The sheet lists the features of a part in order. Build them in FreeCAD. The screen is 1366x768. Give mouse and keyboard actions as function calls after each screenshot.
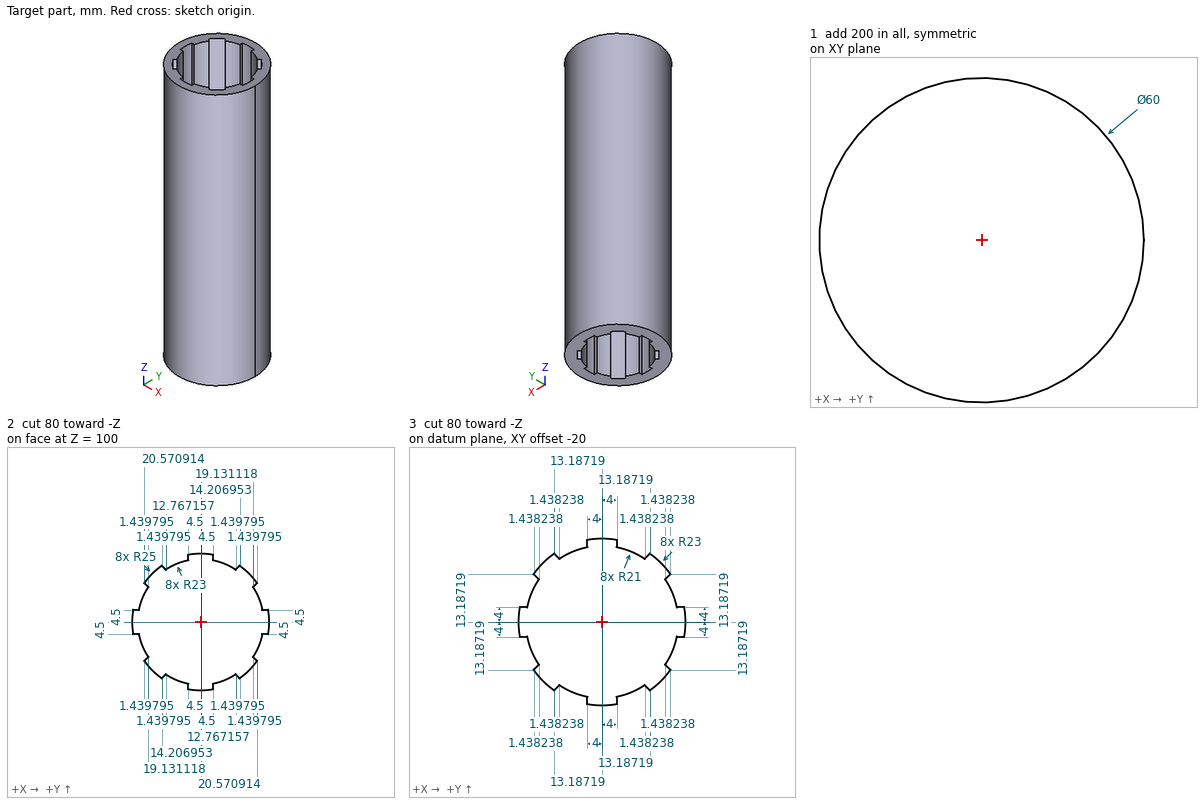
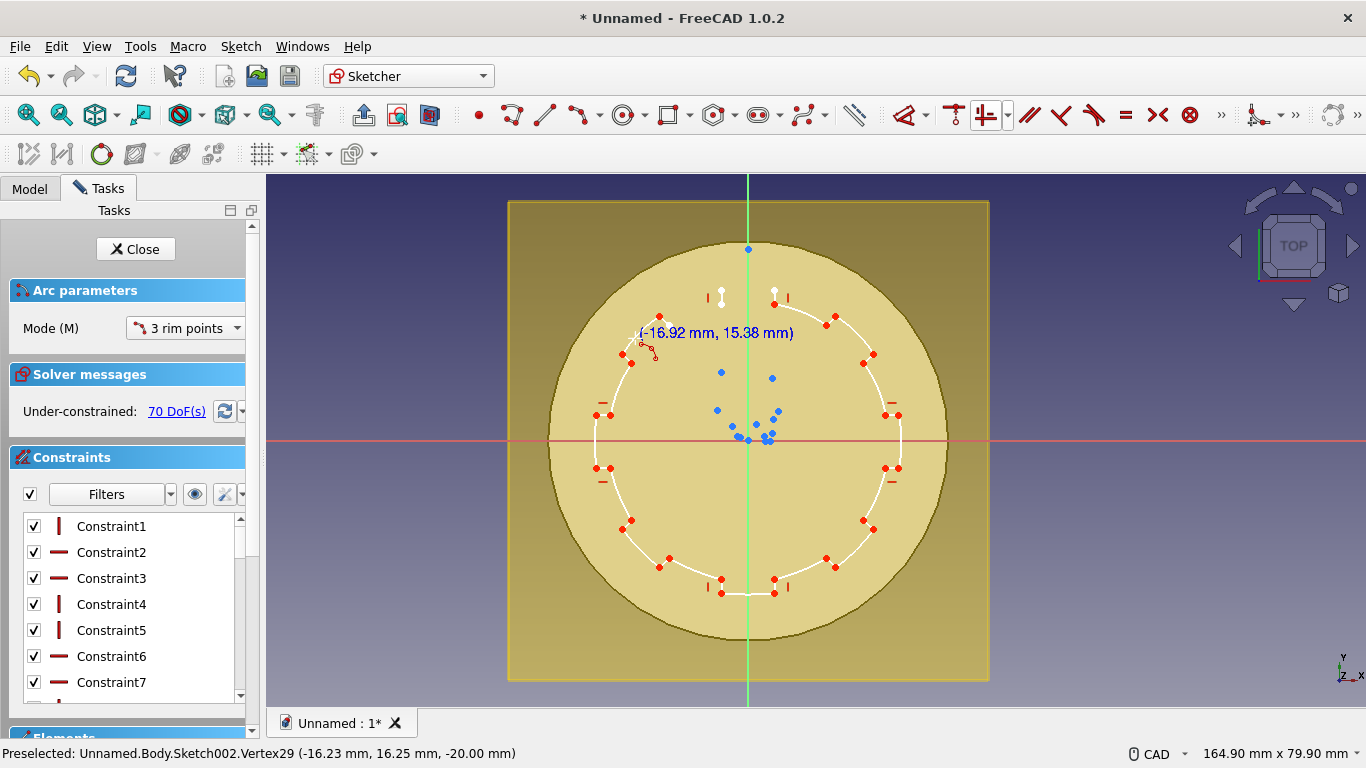
scroll(670, 325, up, 5)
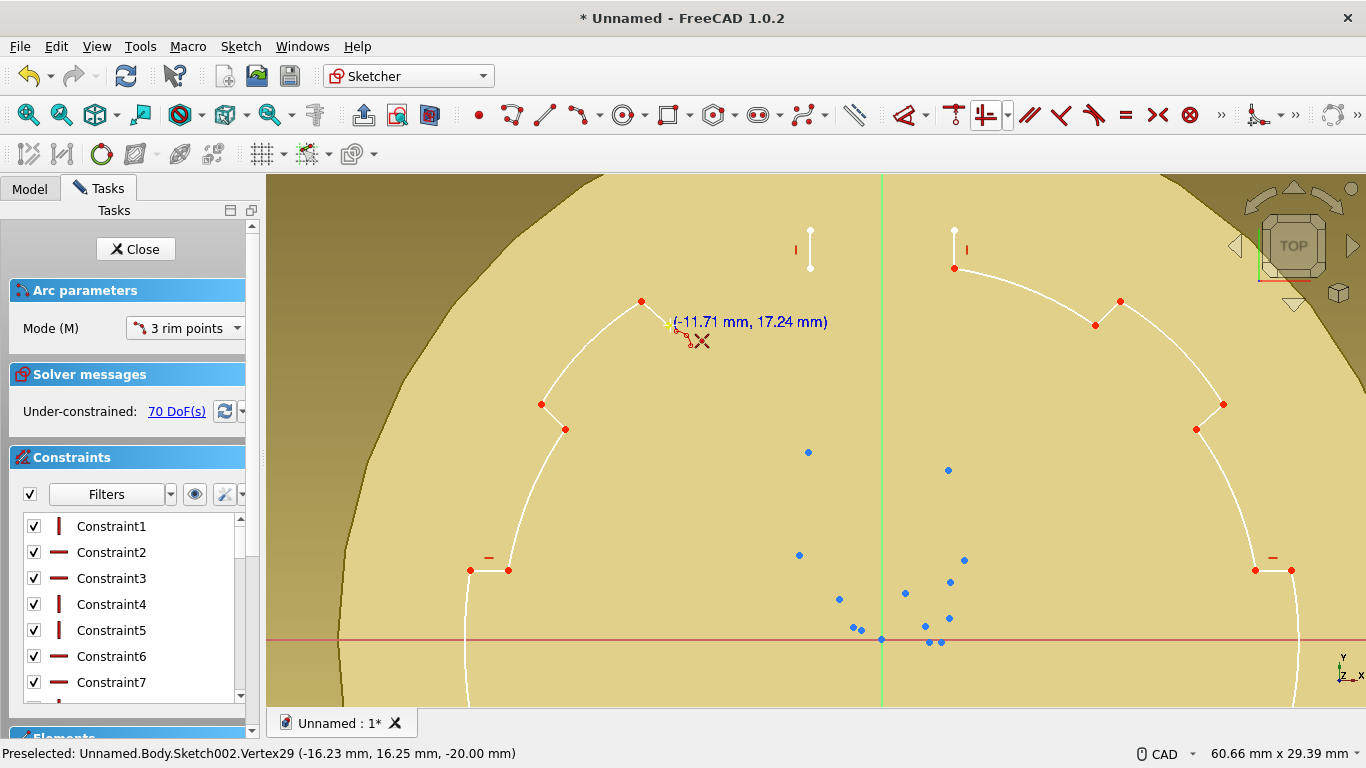
click(669, 326)
click(810, 269)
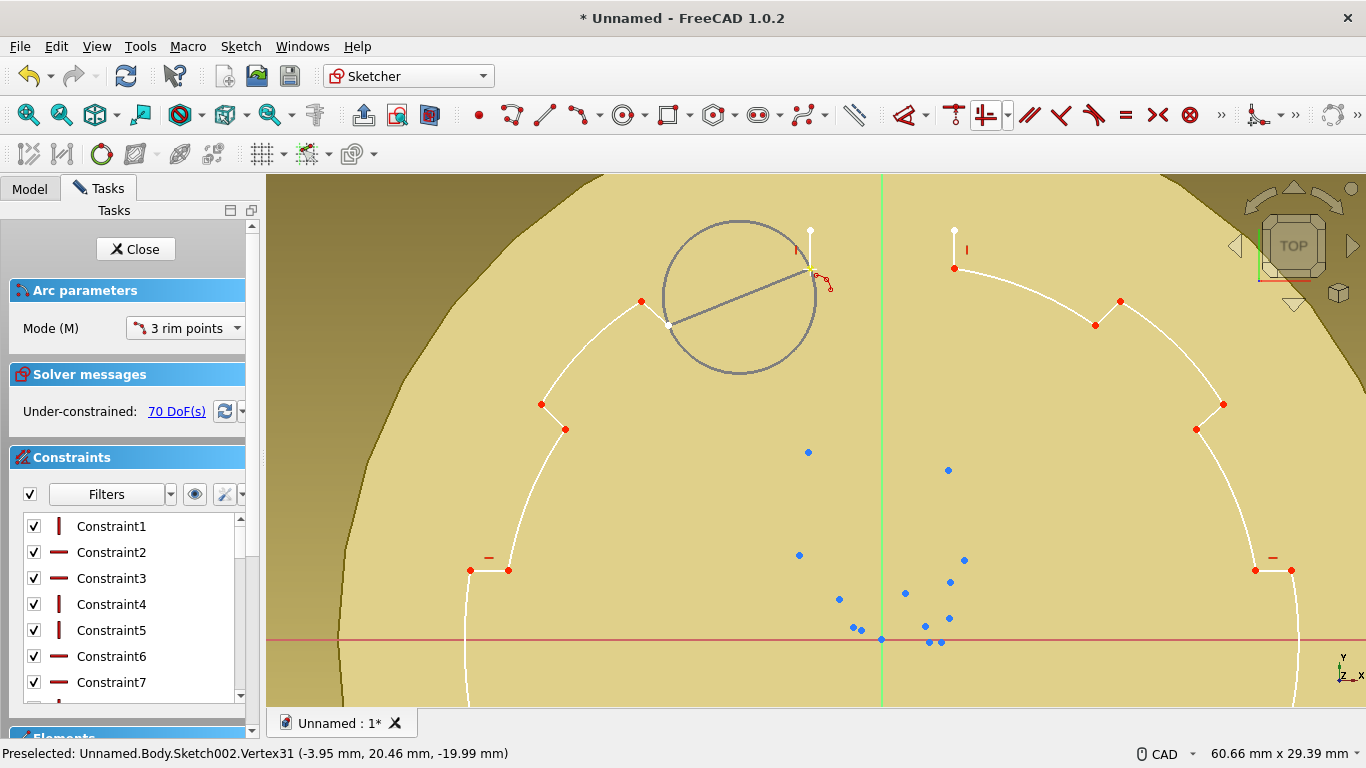
scroll(736, 288, up, 4)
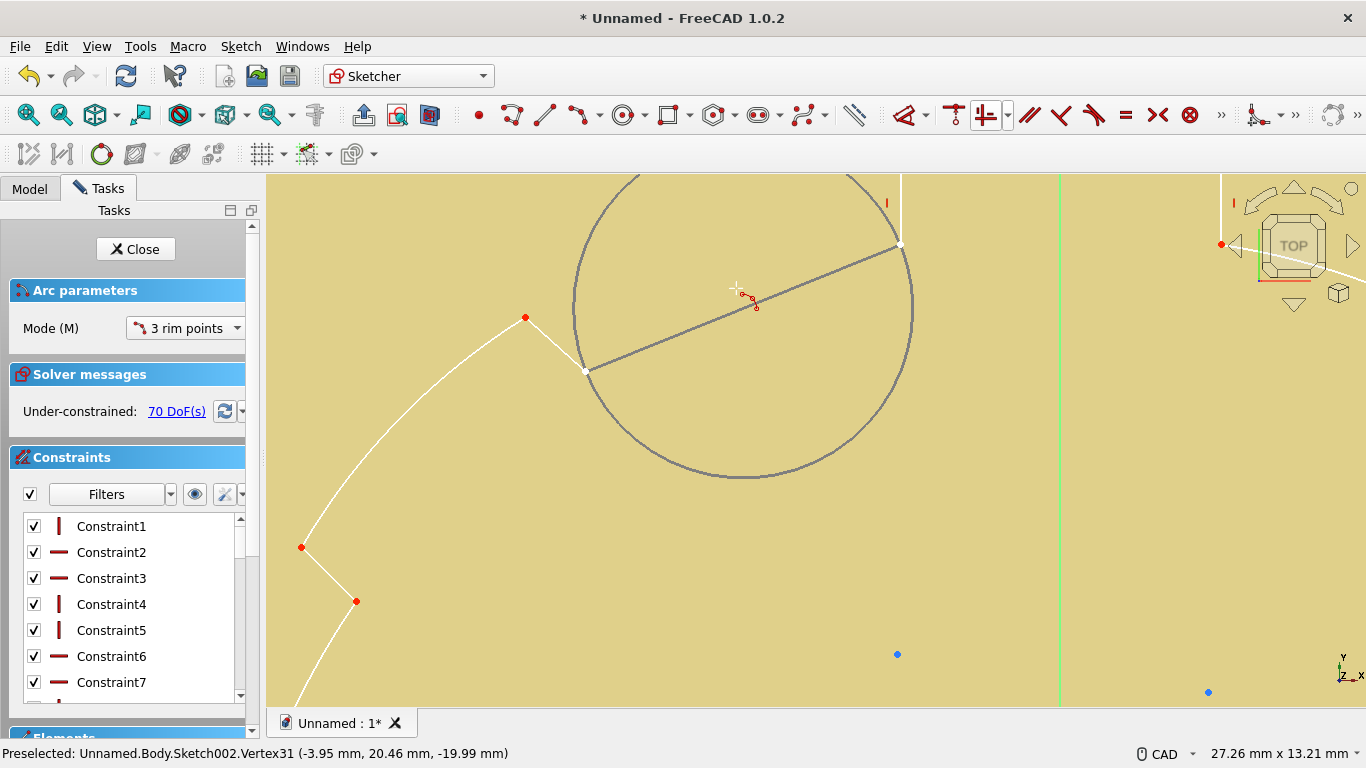
click(736, 288)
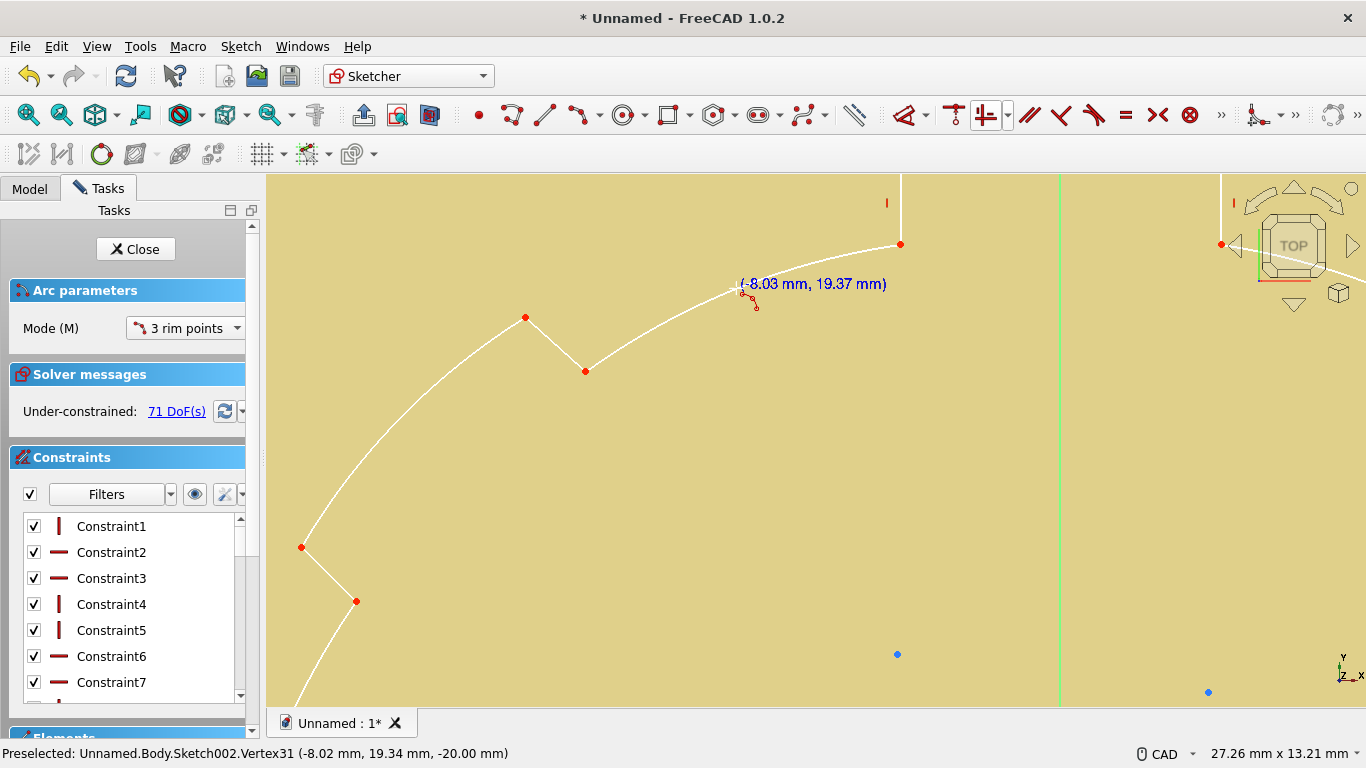
scroll(686, 316, down, 9)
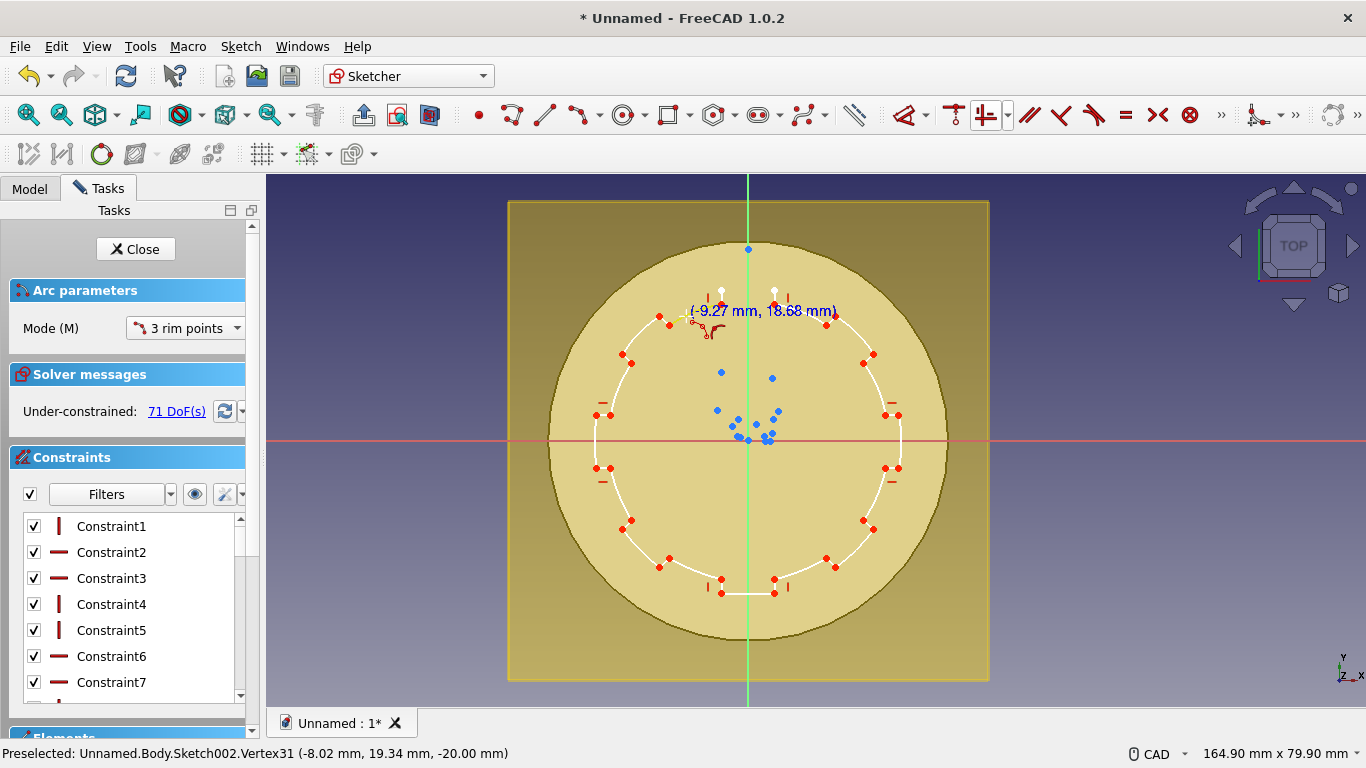
scroll(721, 290, up, 5)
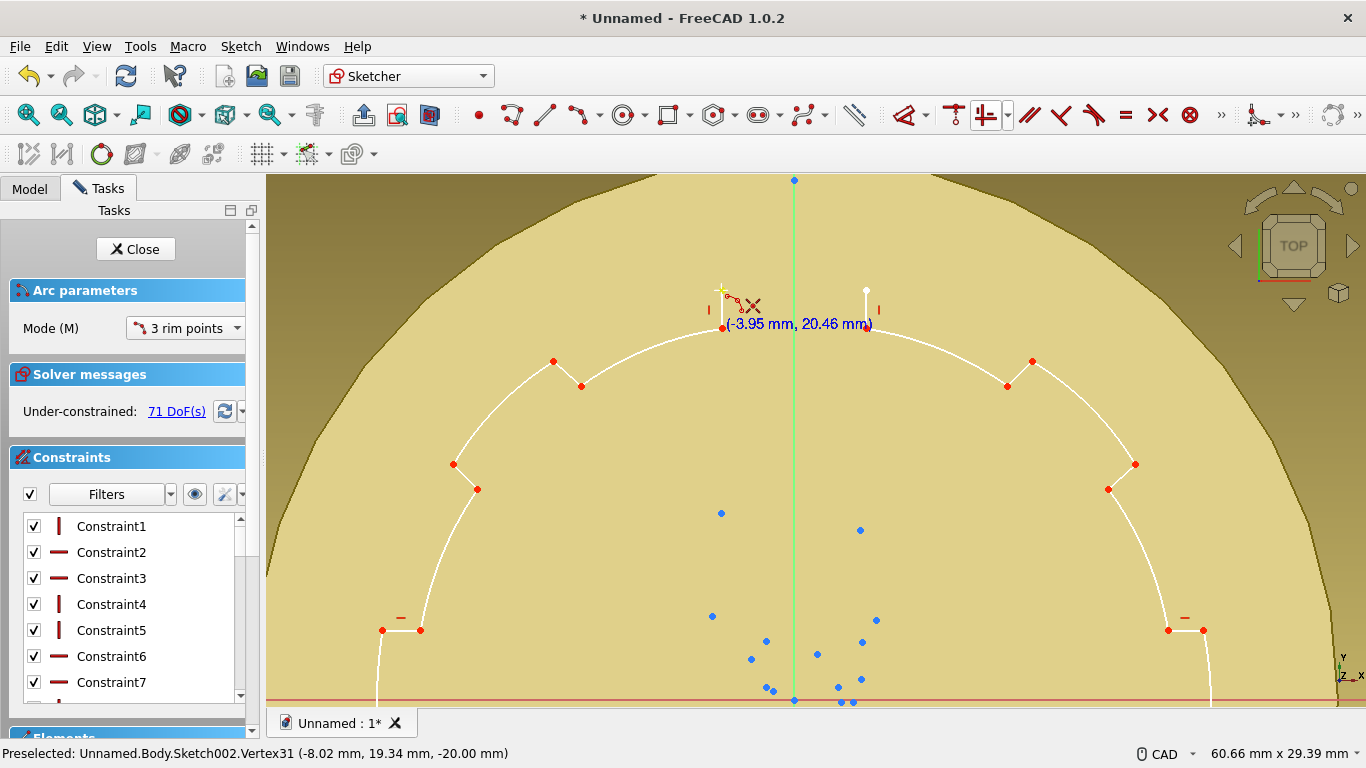
click(722, 291)
click(866, 291)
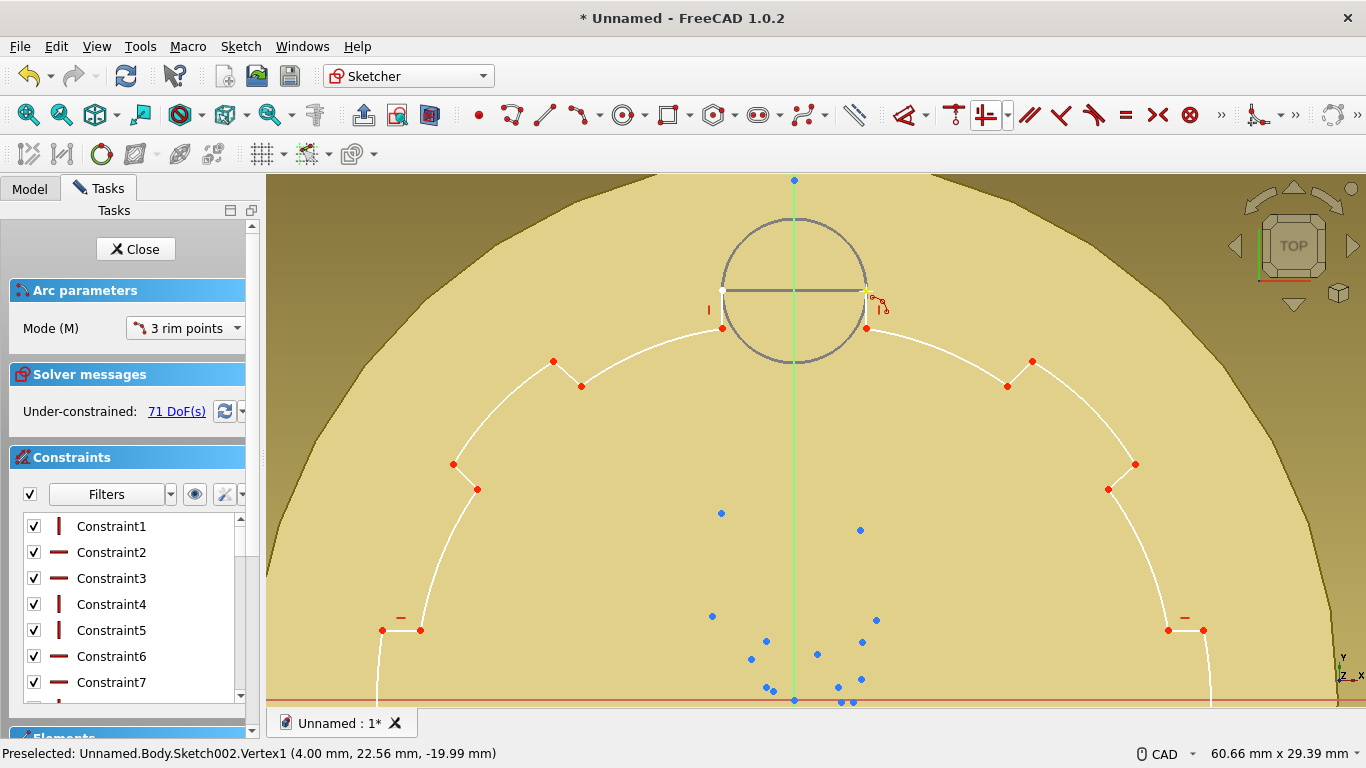
scroll(809, 283, up, 5)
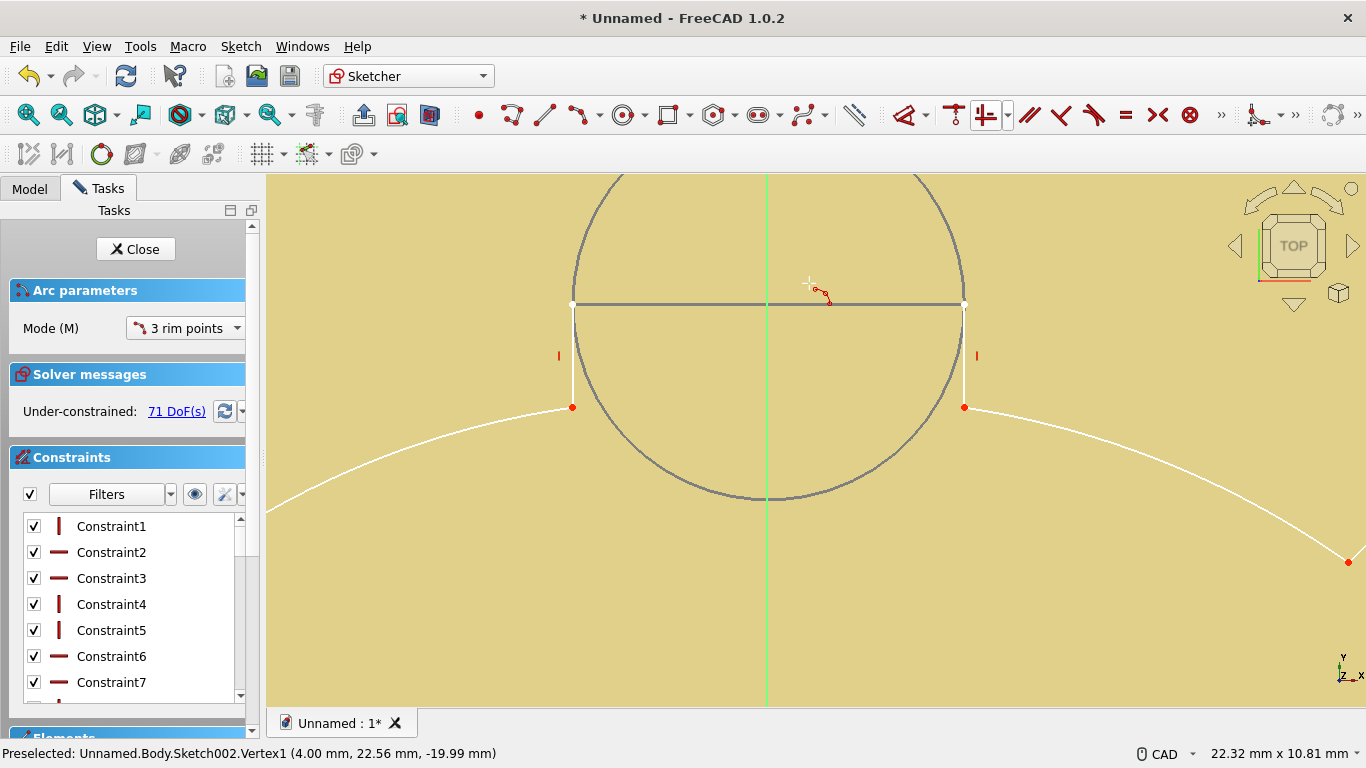
click(807, 283)
key(Escape)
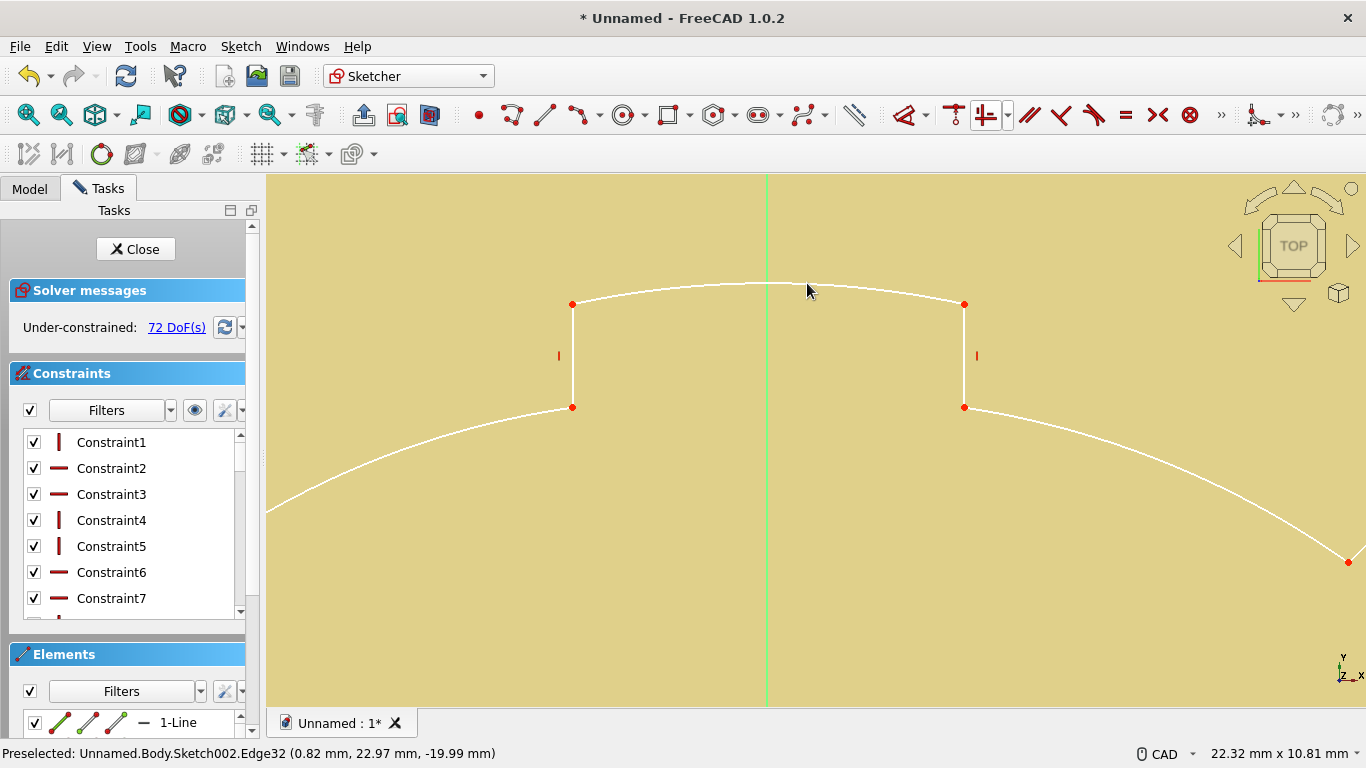
scroll(744, 288, down, 10)